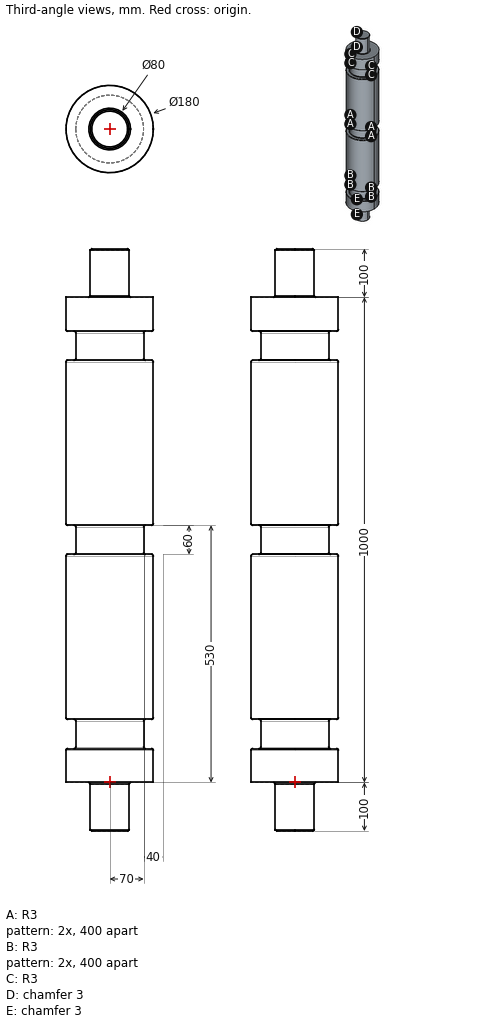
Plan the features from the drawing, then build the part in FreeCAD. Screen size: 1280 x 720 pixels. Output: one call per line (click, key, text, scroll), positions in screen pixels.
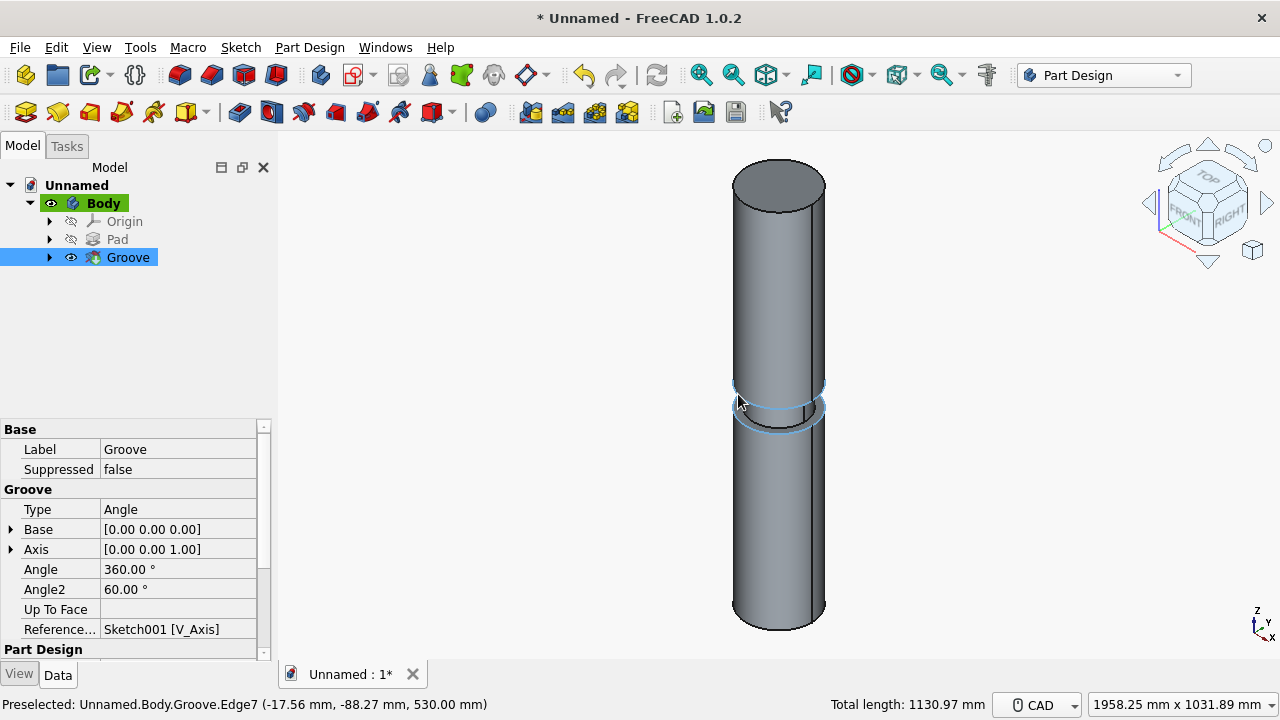
key(2)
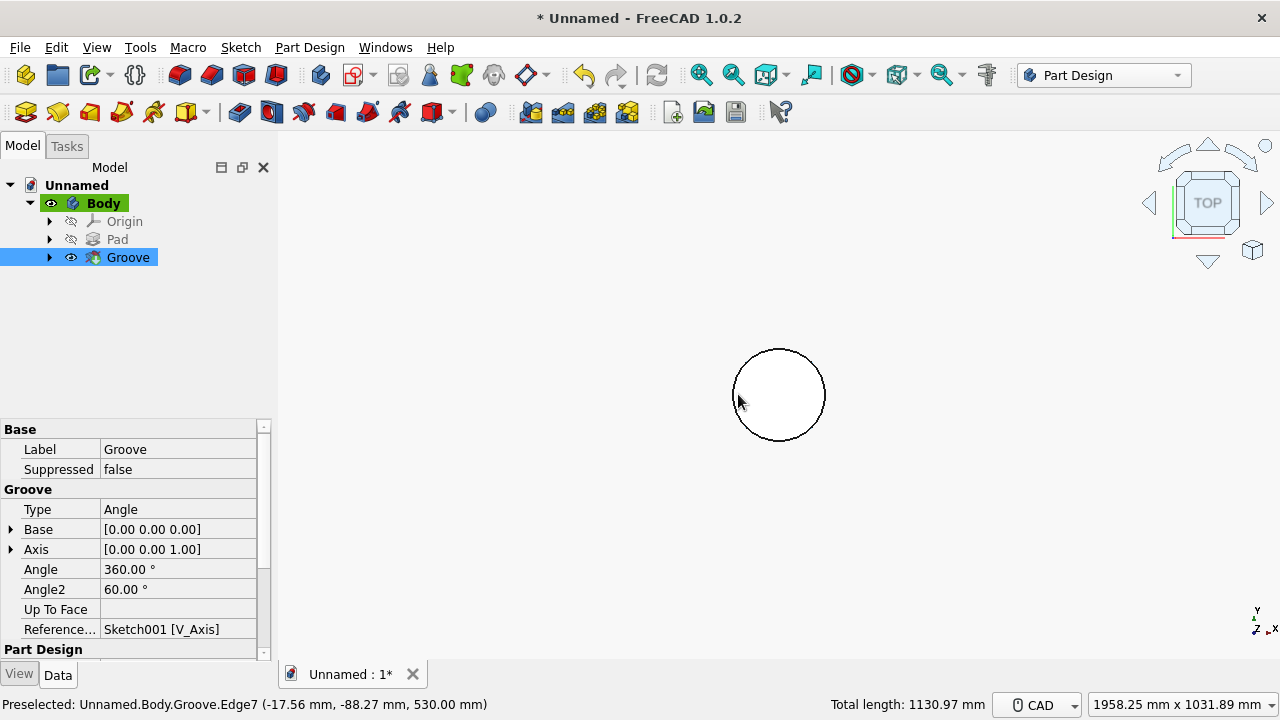
click(702, 76)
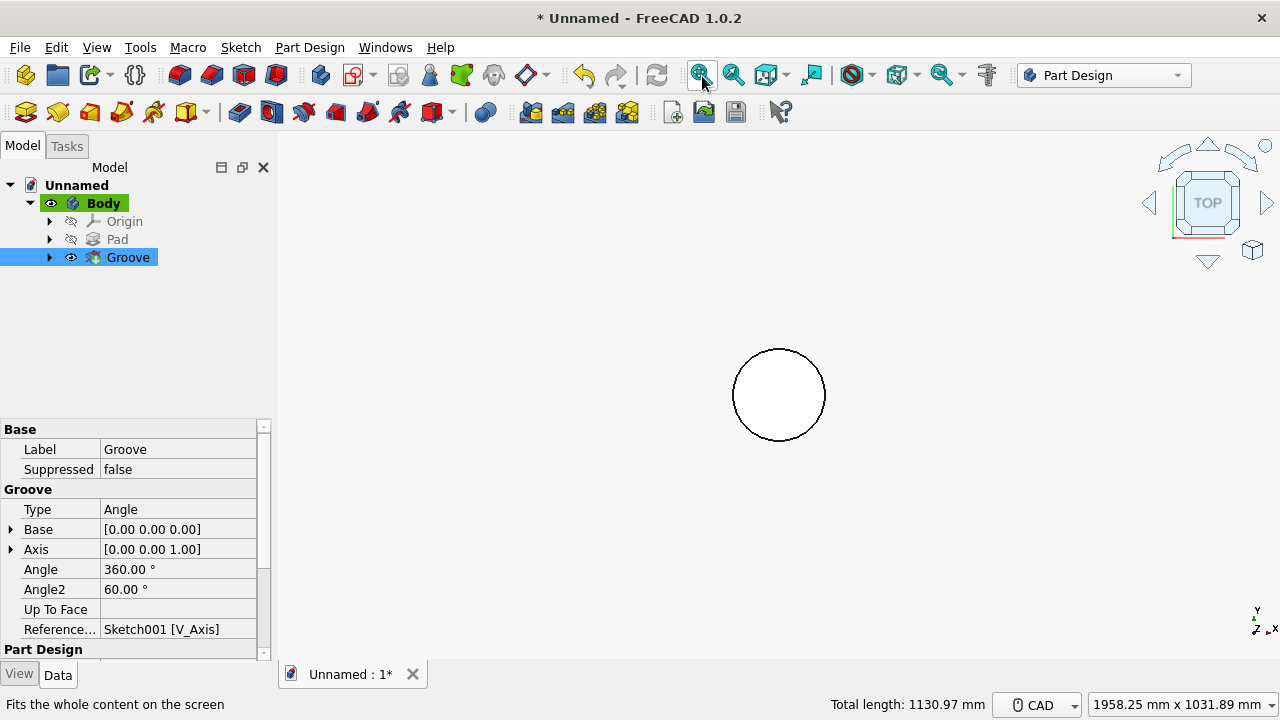
key(1)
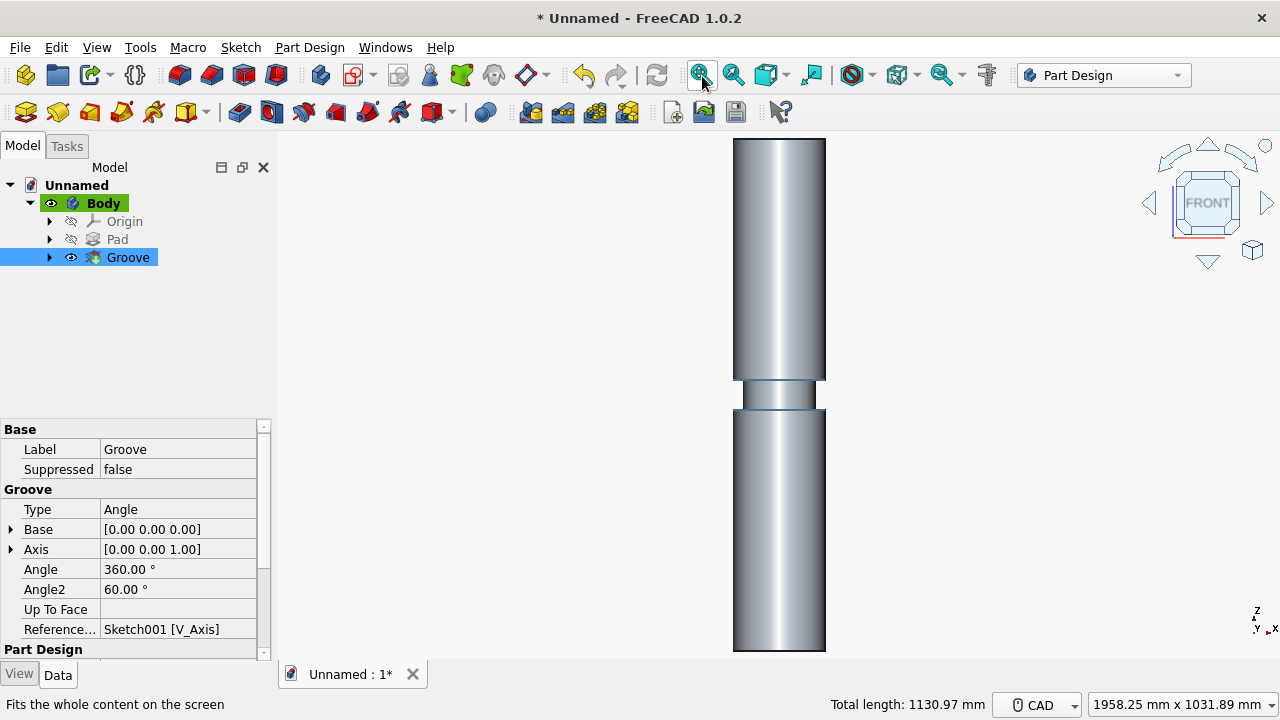
key(3)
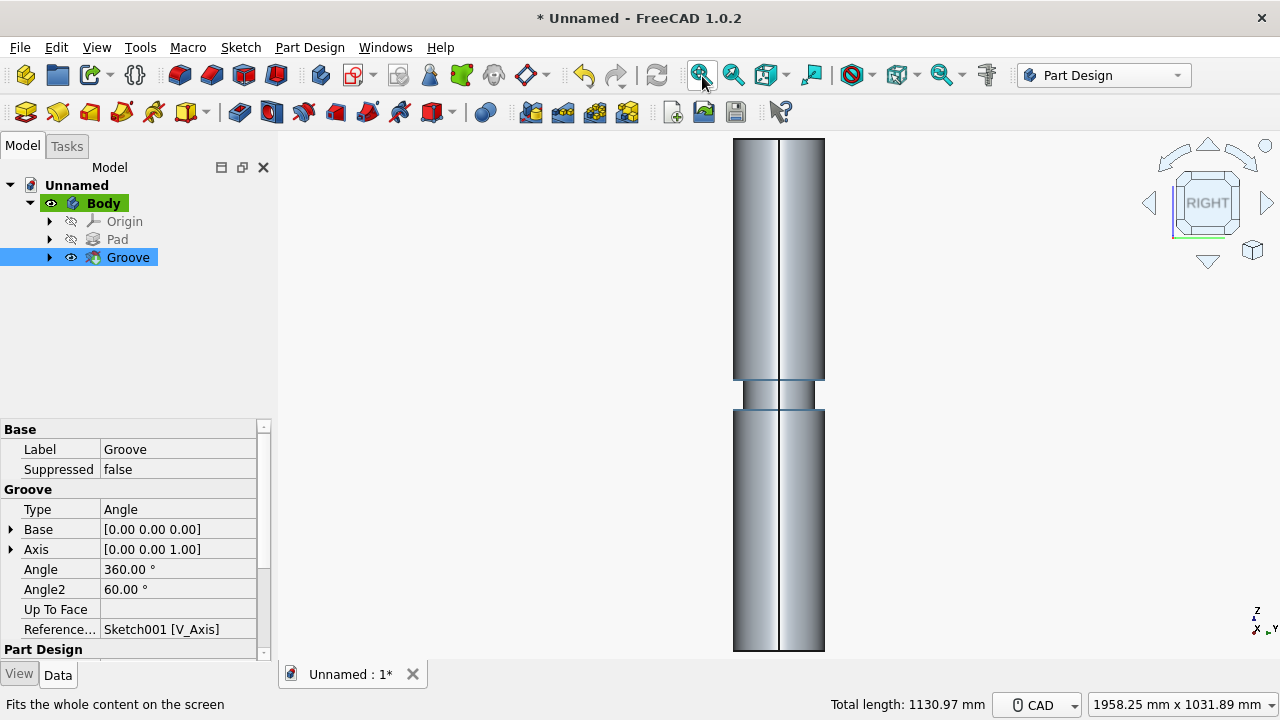
key(5)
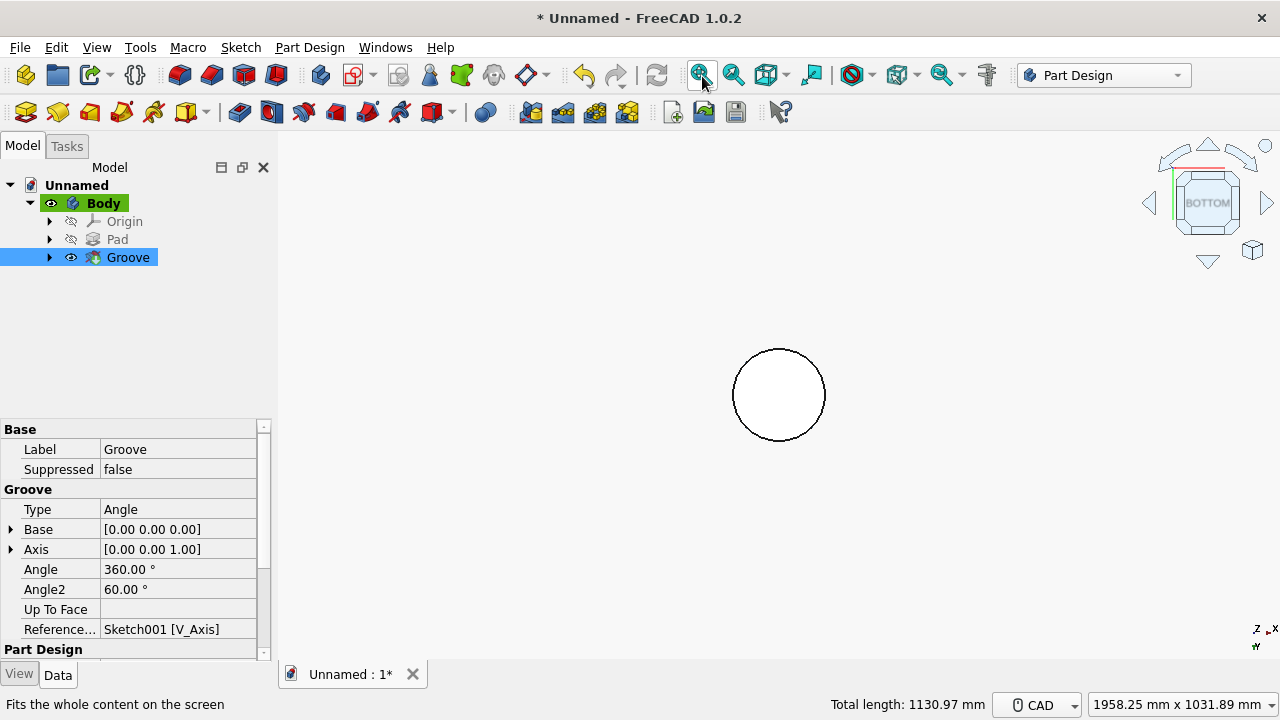
click(702, 76)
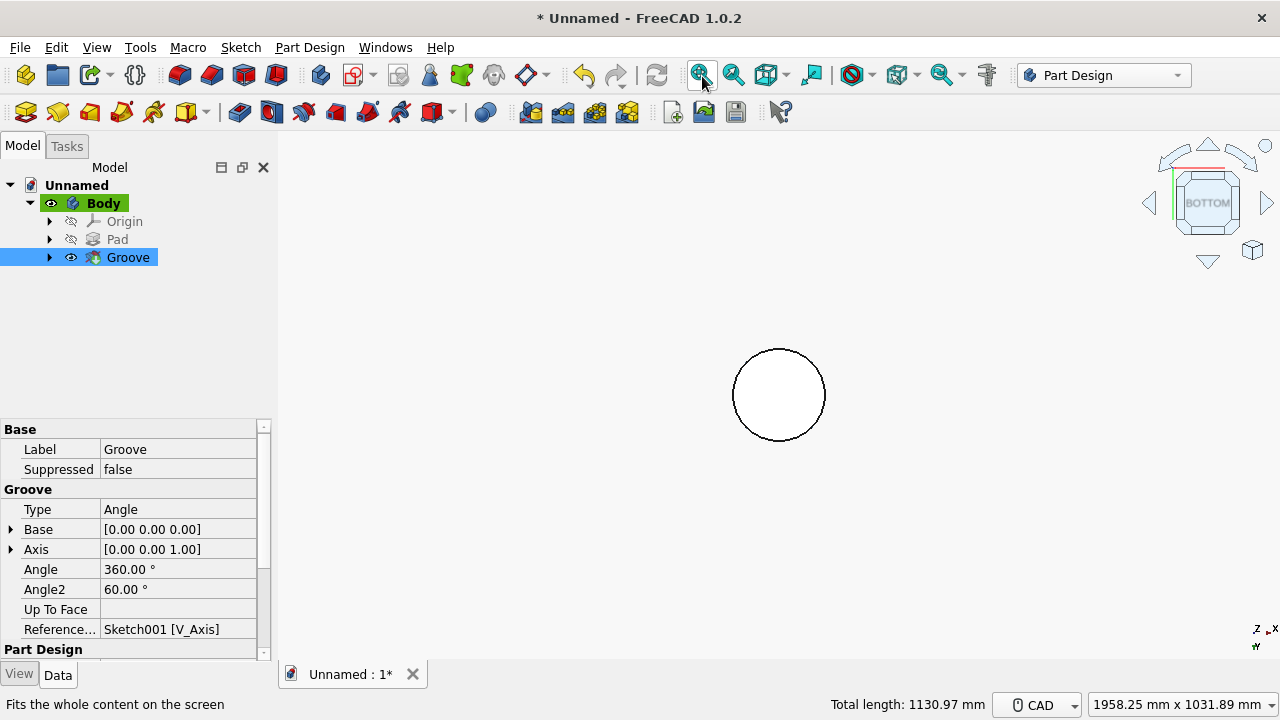
key(4)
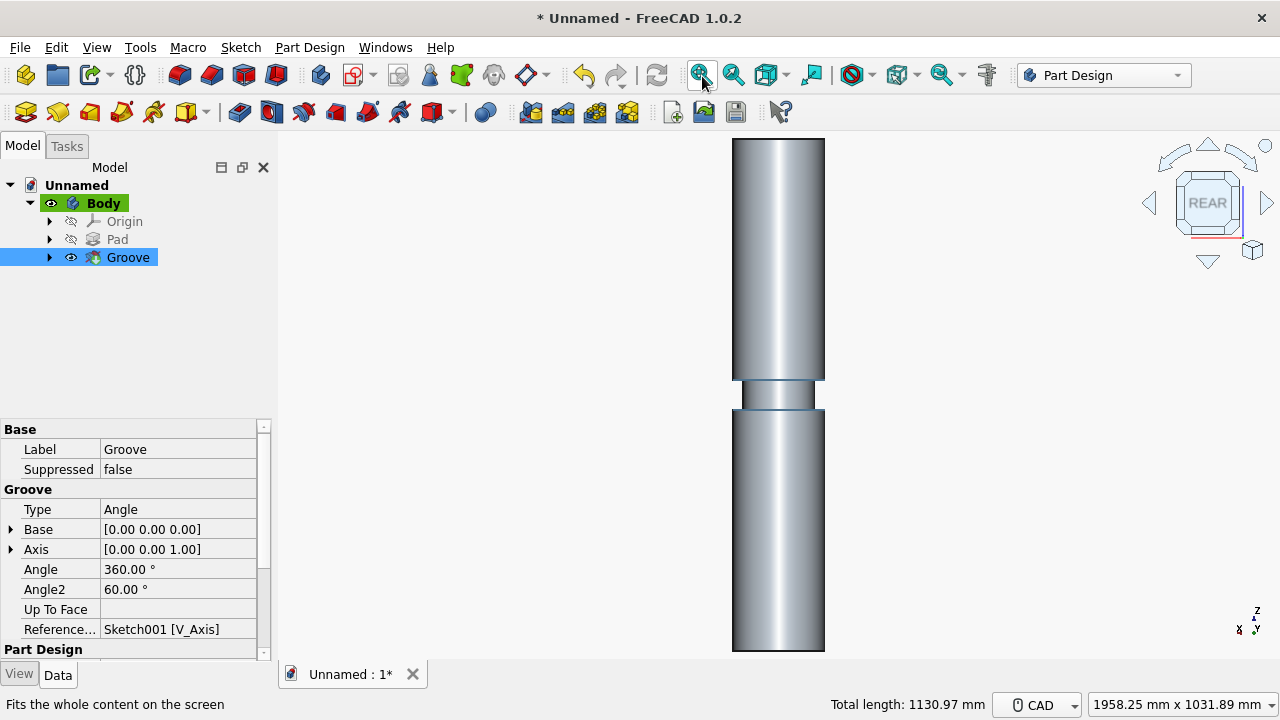
key(6)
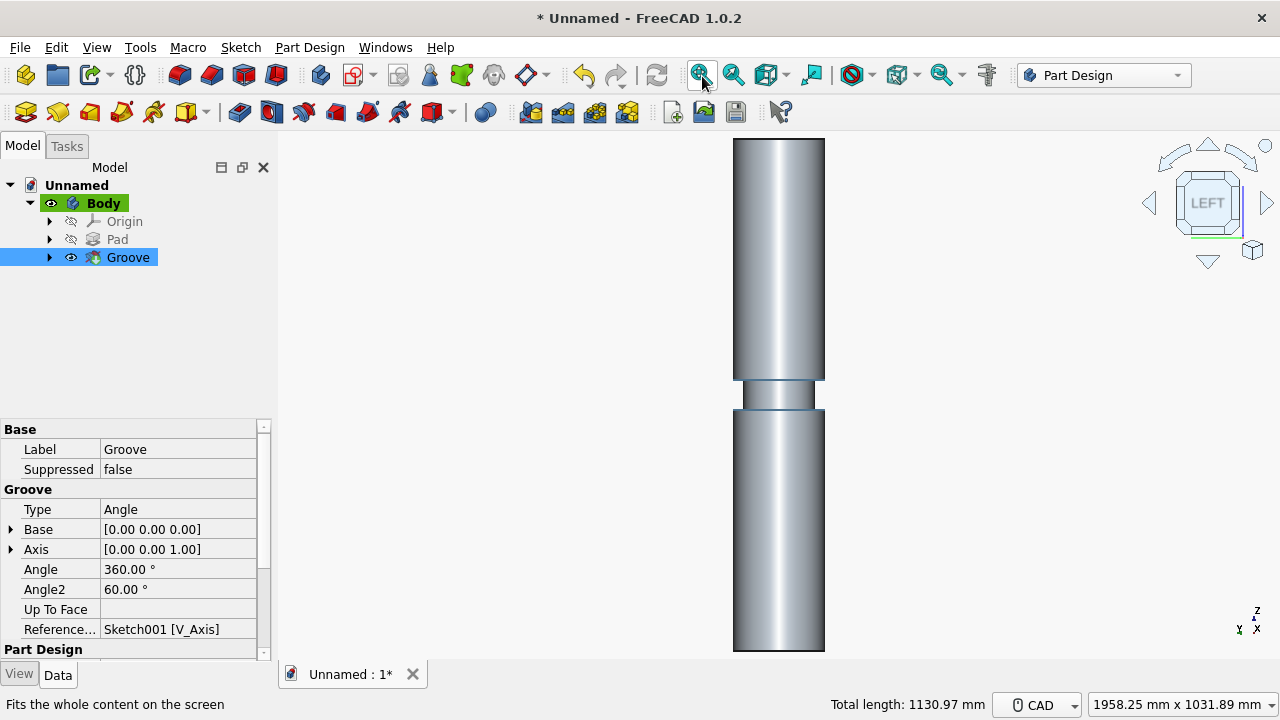
key(v)
key(3)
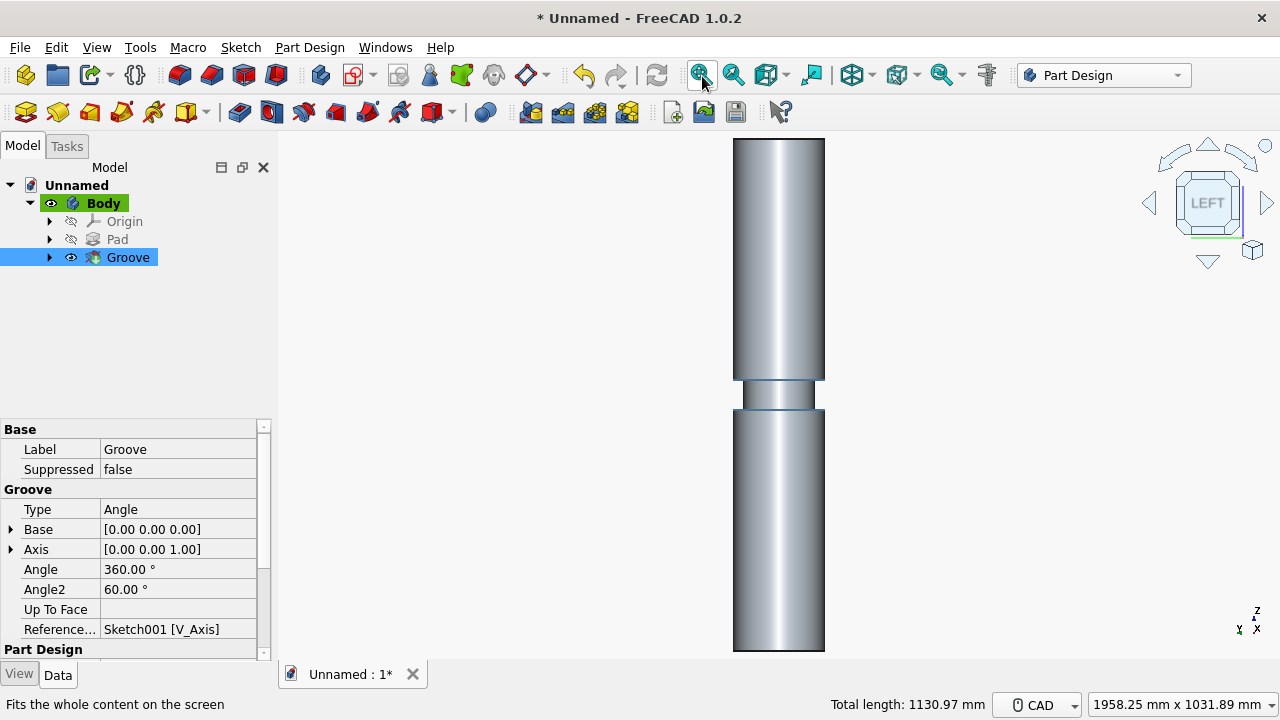
key(0)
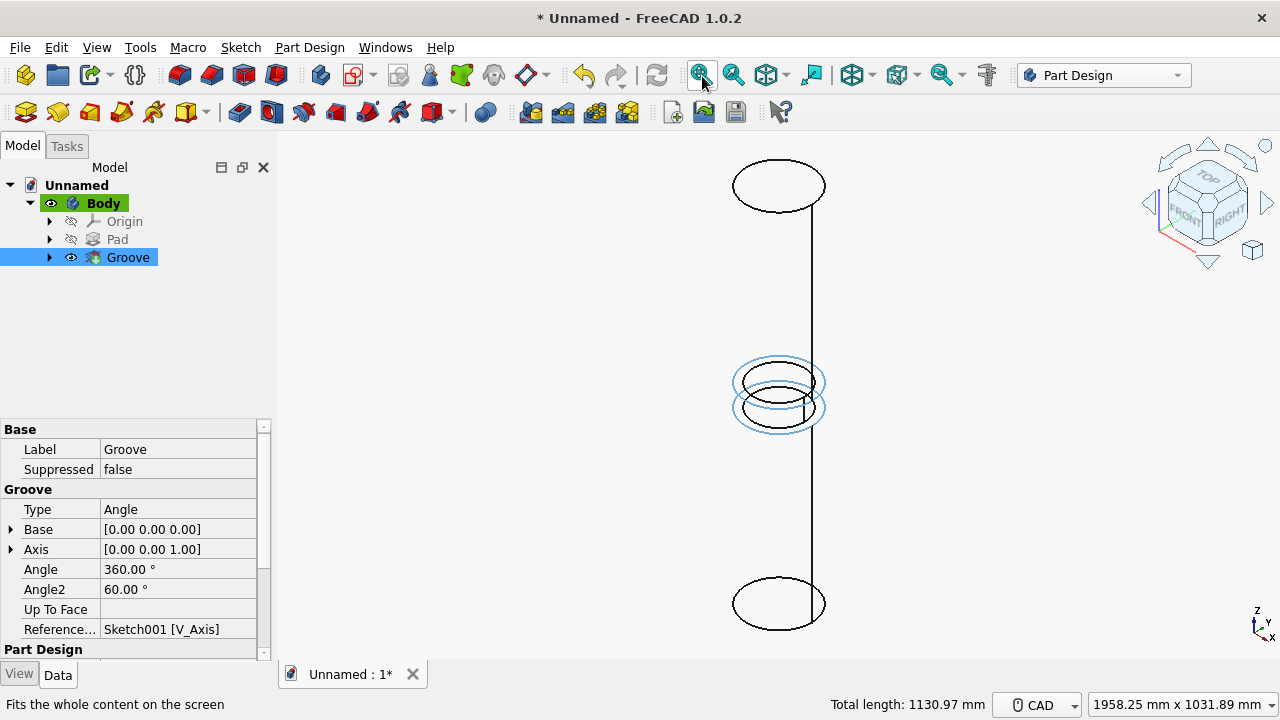
click(754, 367, ctrl)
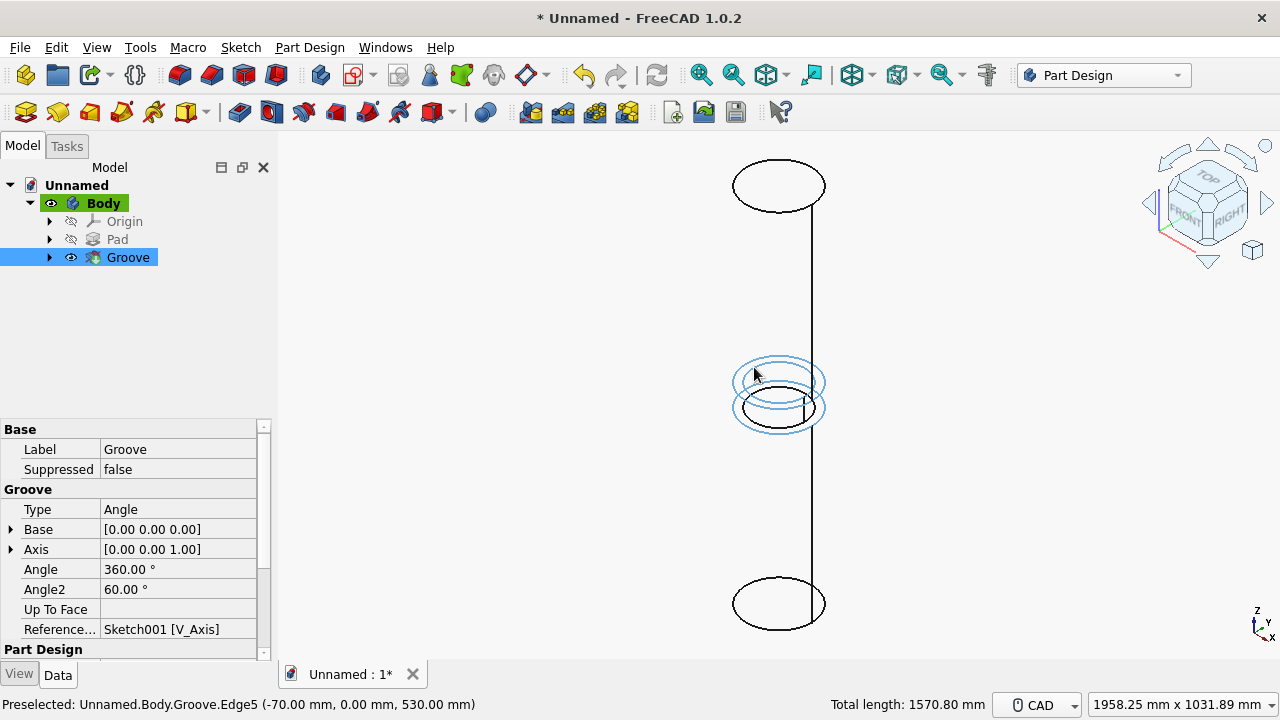
click(773, 386, ctrl)